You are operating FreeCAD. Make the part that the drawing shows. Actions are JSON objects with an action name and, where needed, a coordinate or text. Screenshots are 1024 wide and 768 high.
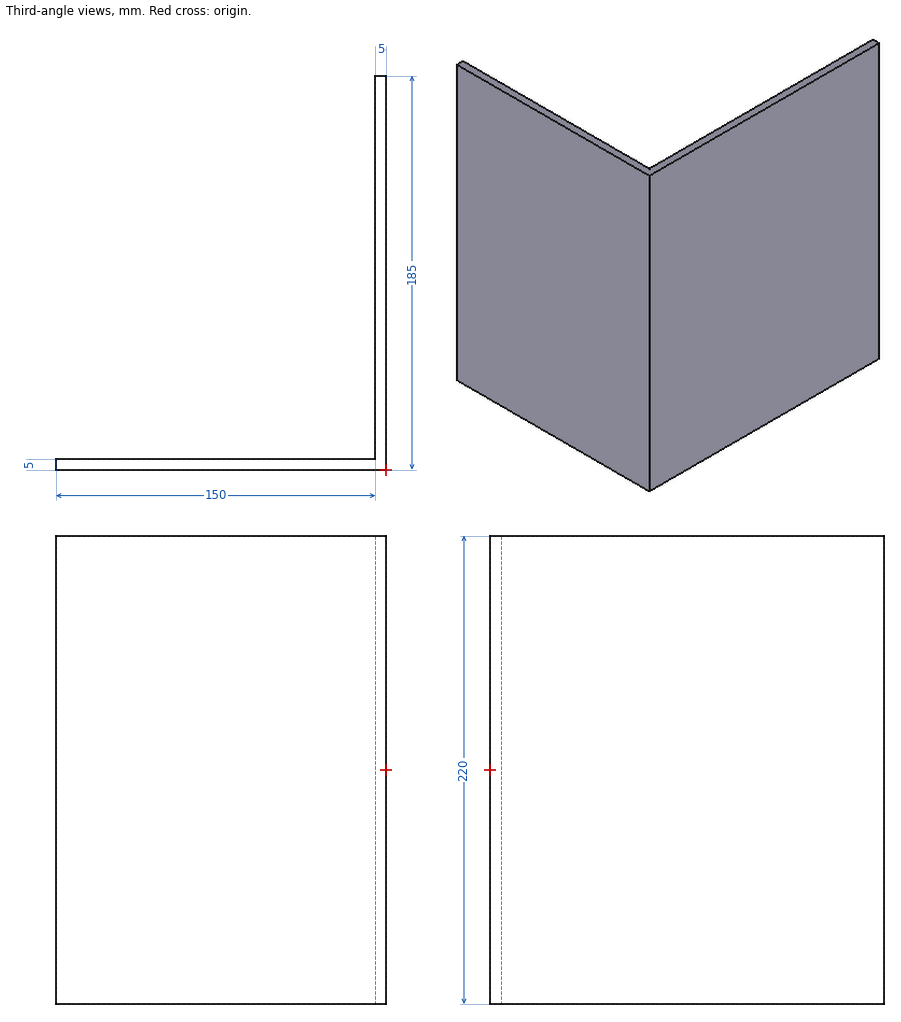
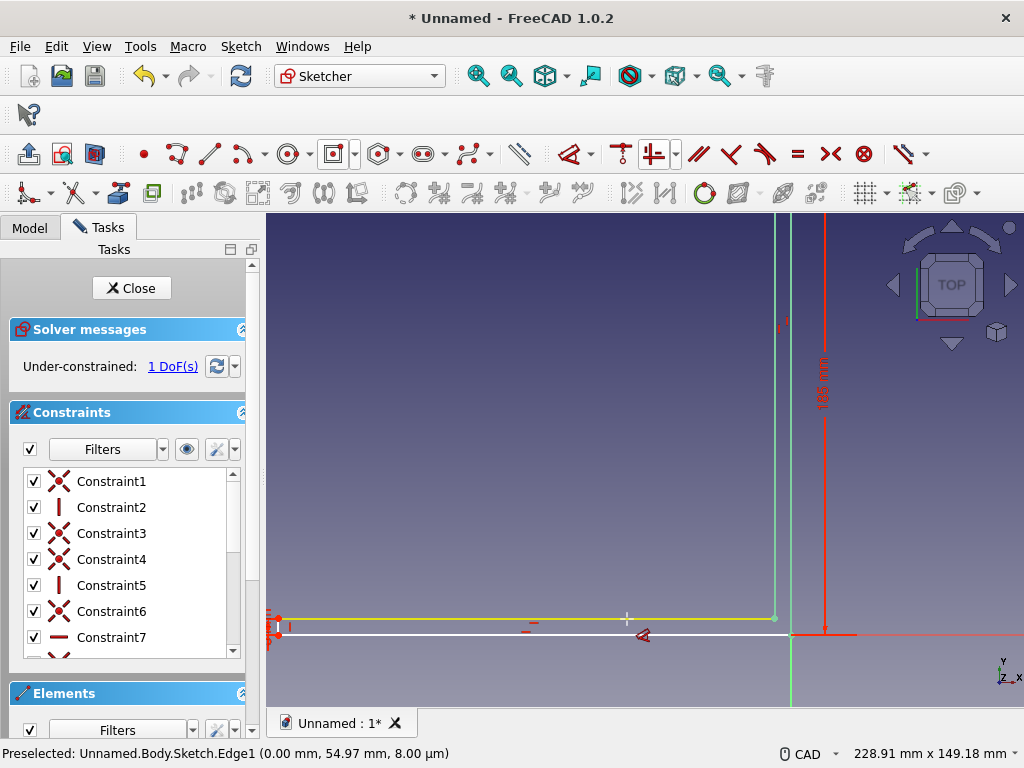
{"action": "left_click", "coordinate": [626, 619]}
{"action": "left_click", "coordinate": [534, 653]}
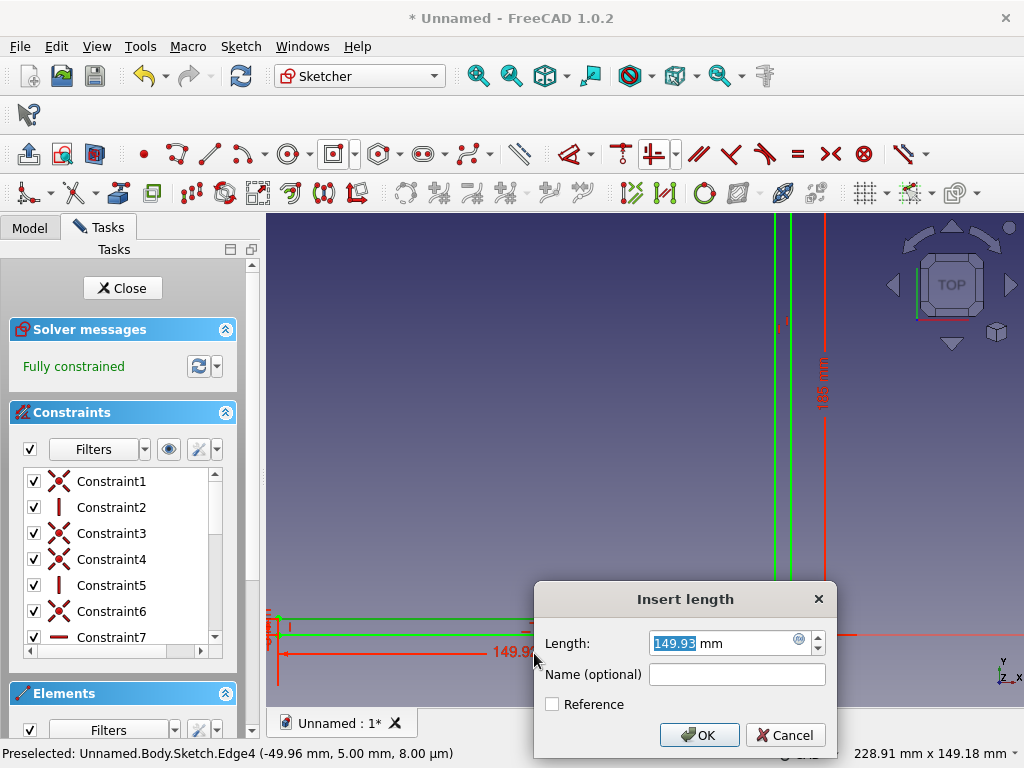
{"action": "type", "text": "150"}
{"action": "key", "text": "Return"}
{"action": "key", "text": "Escape"}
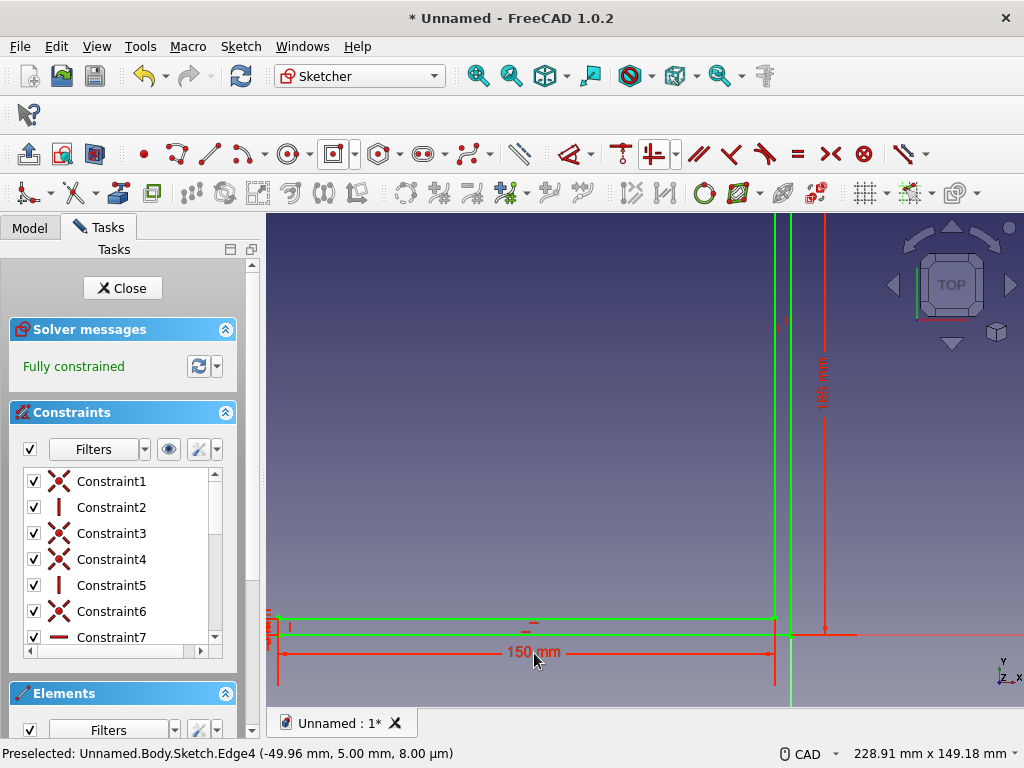
{"action": "left_click", "coordinate": [123, 288]}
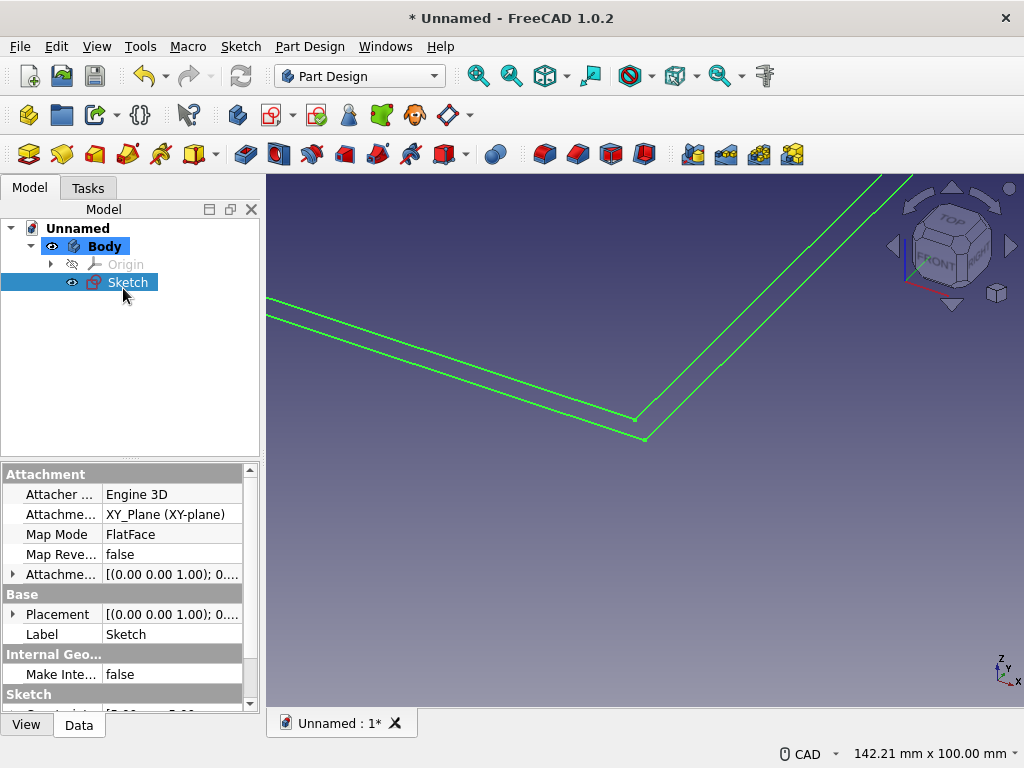
{"action": "left_click", "coordinate": [29, 154]}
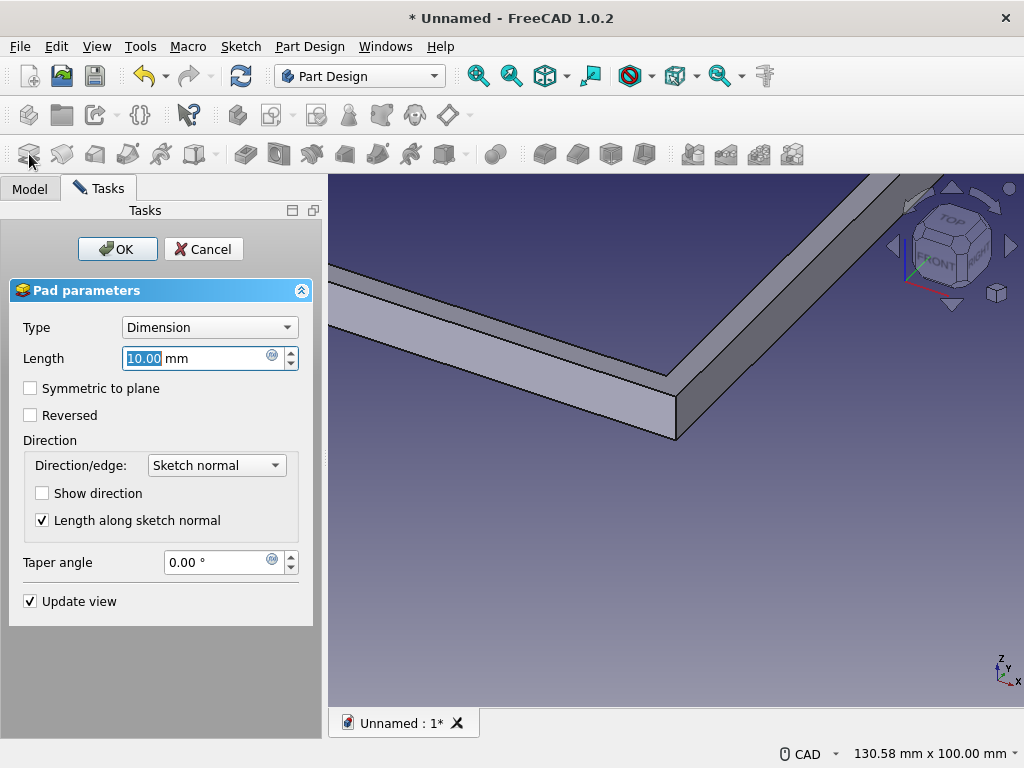
{"action": "type", "text": "220"}
{"action": "key", "text": "Tab"}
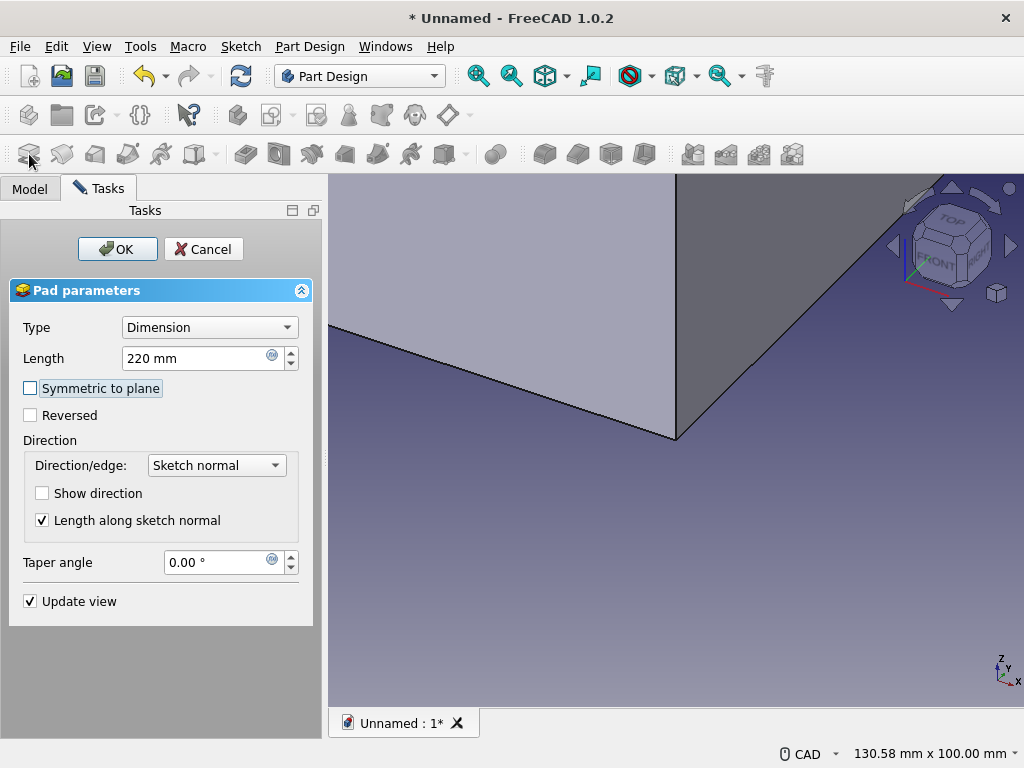
{"action": "left_click", "coordinate": [31, 388]}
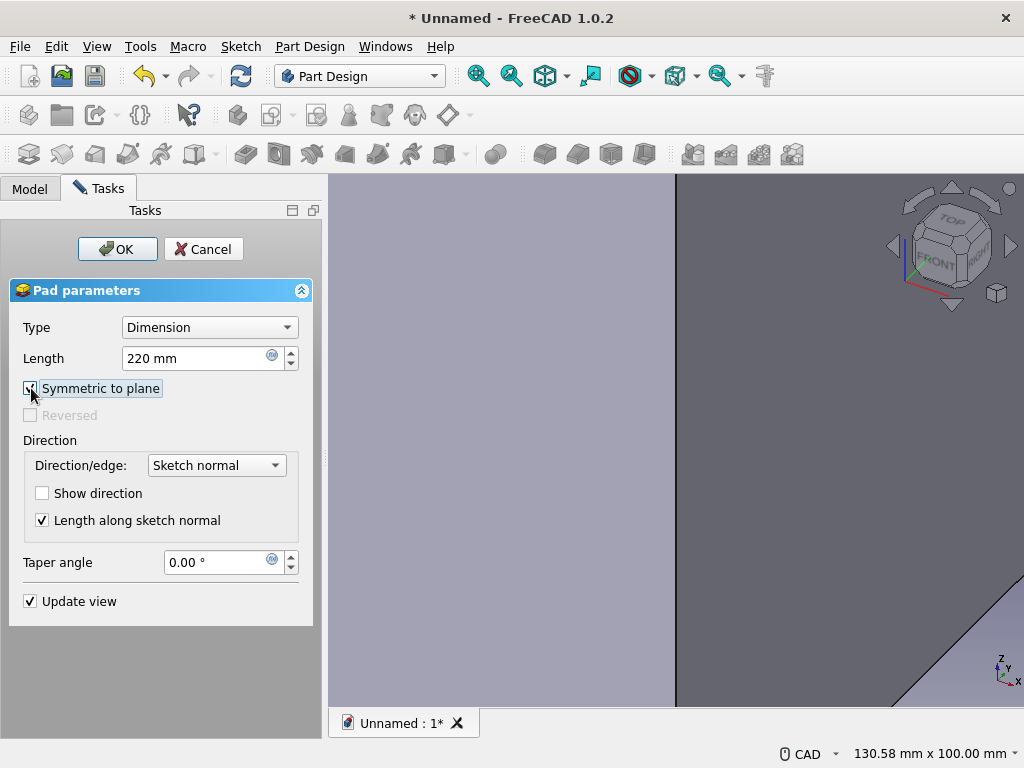
{"action": "left_click", "coordinate": [118, 249]}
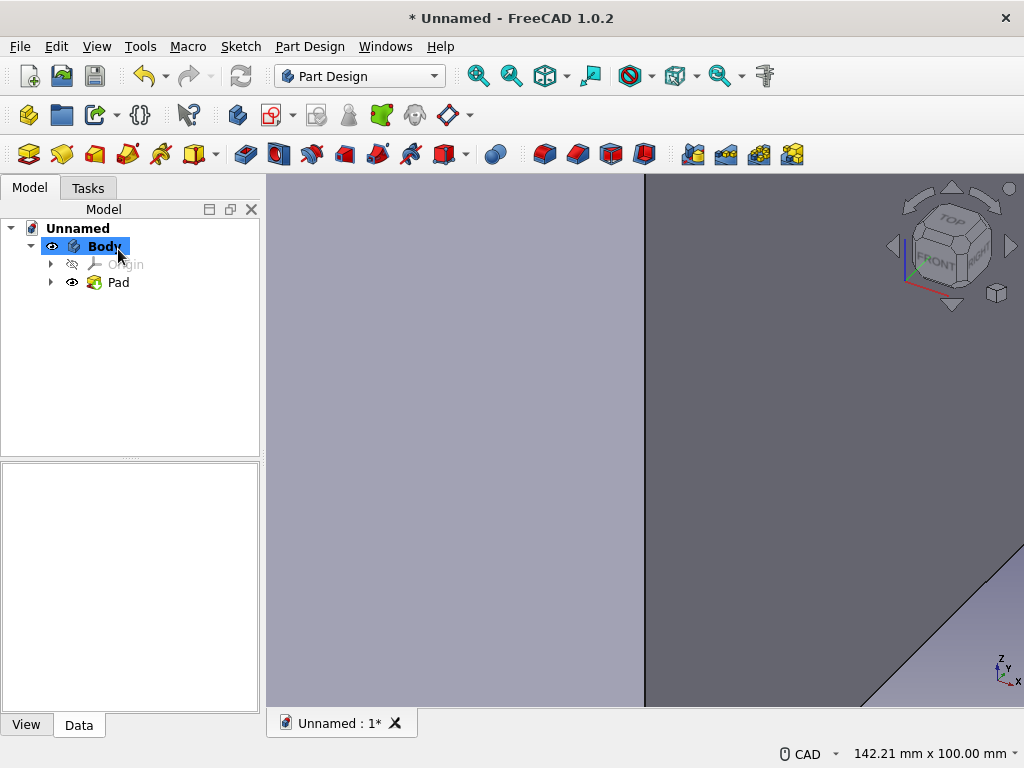
{"action": "key", "text": "0"}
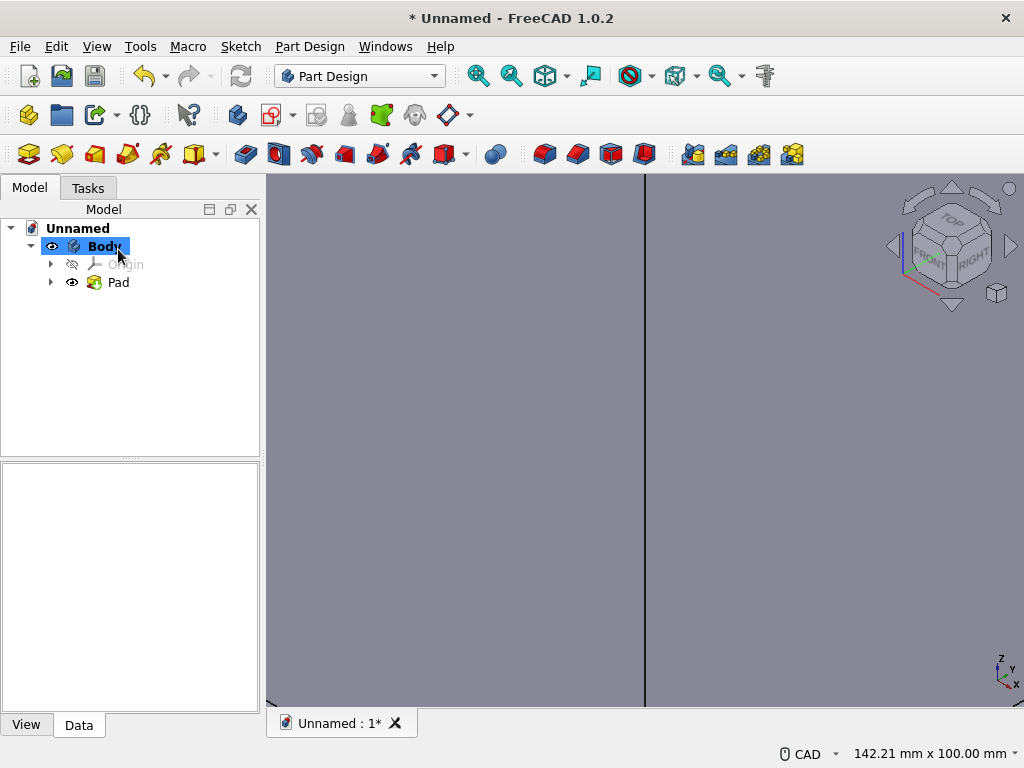
{"action": "left_click", "coordinate": [479, 76]}